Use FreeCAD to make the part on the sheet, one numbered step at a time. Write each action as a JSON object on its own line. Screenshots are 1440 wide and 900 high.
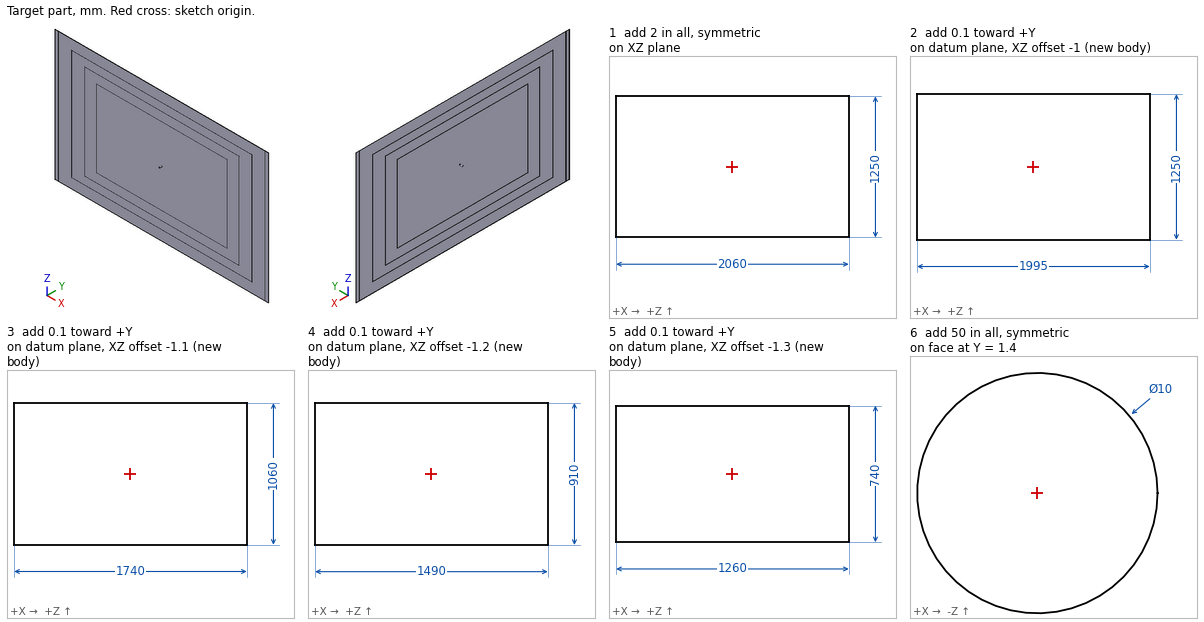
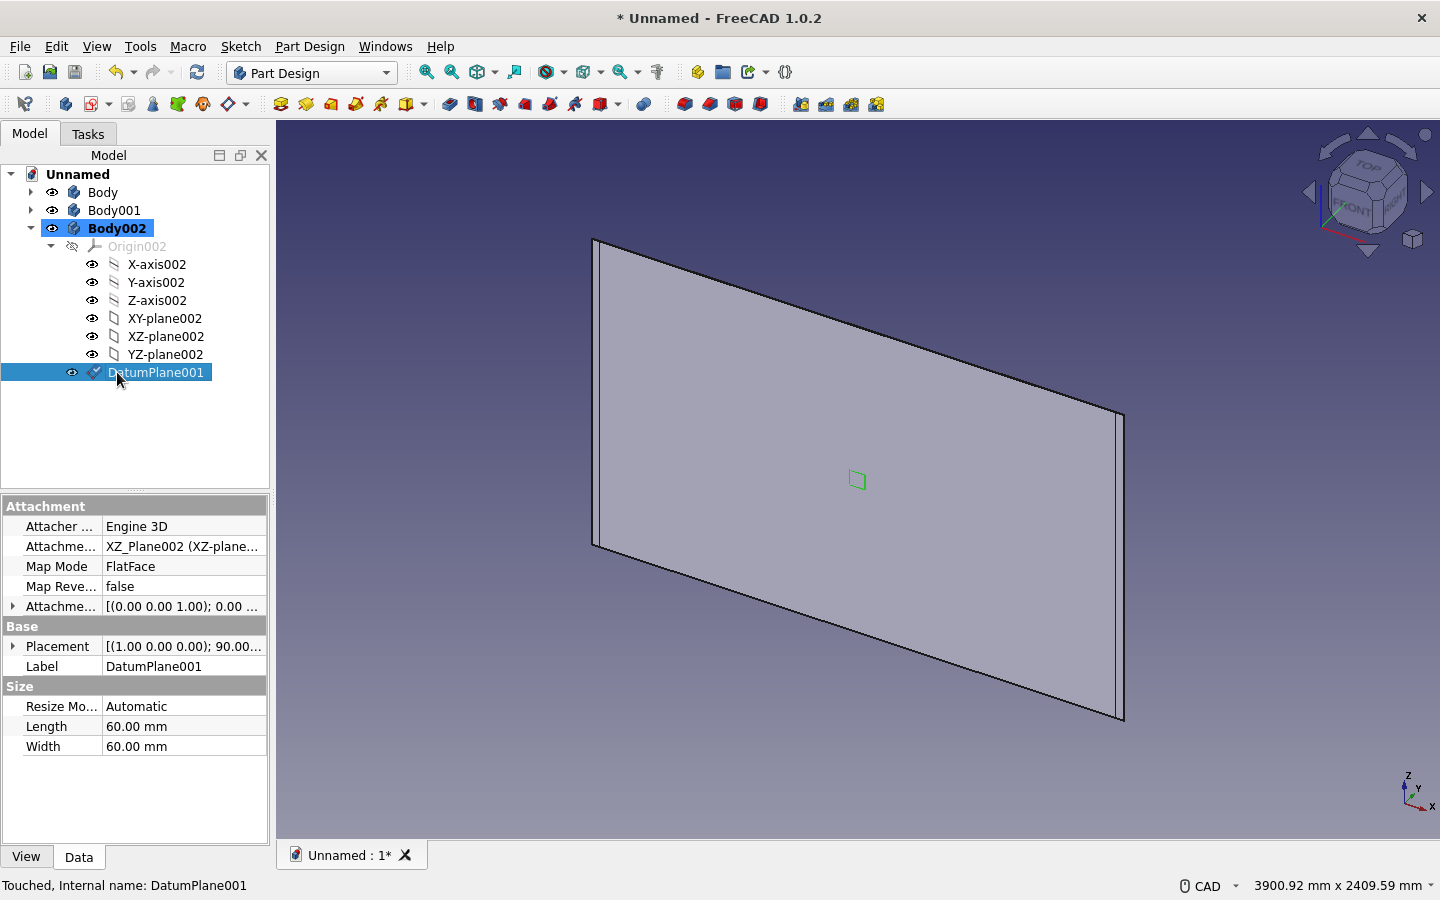
{"action": "left_click", "coordinate": [90, 104]}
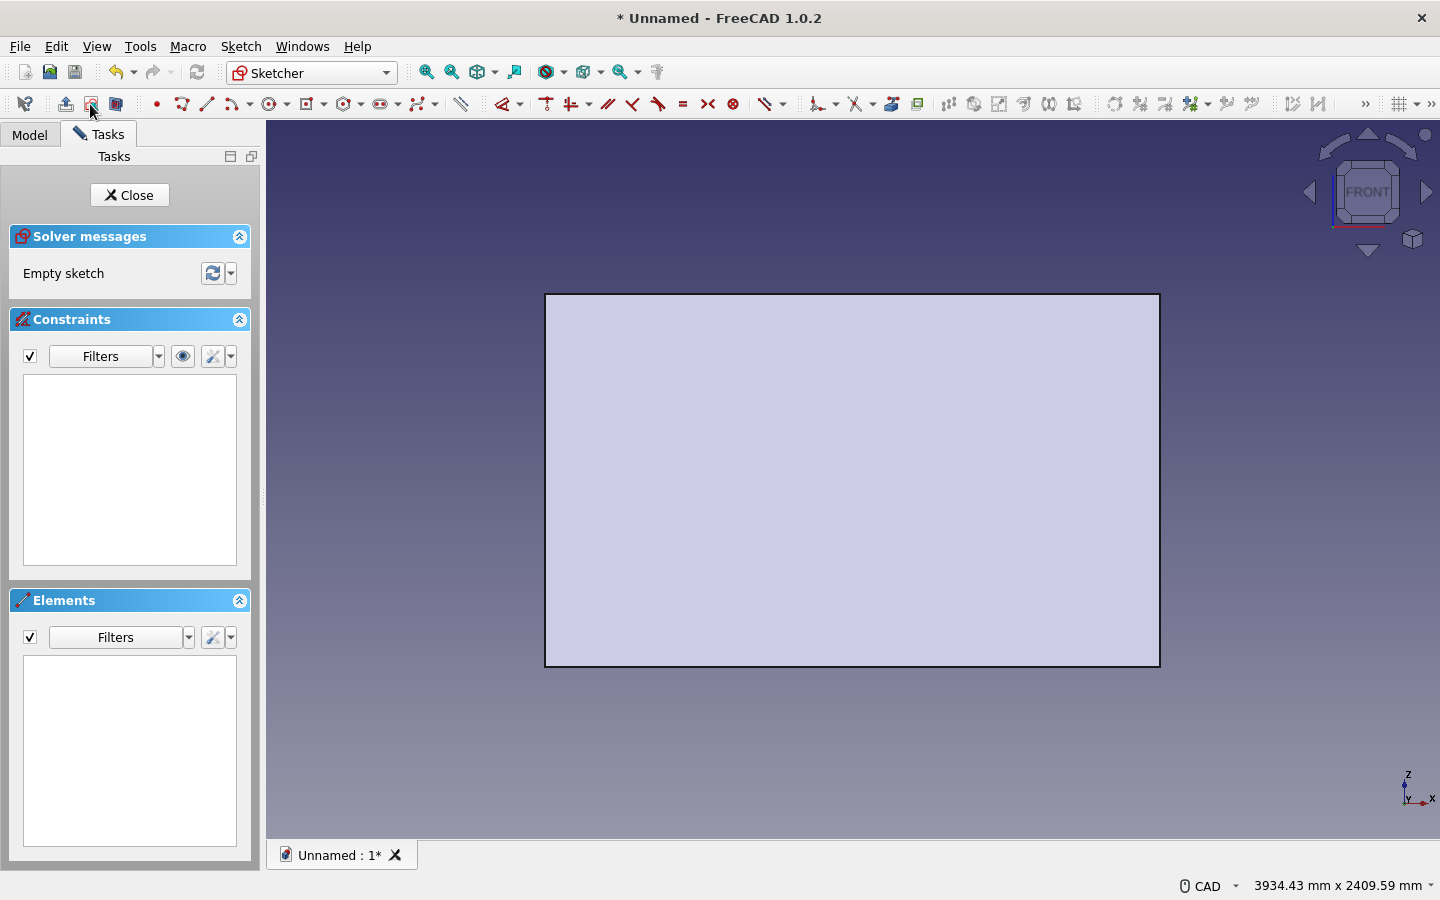
{"action": "left_click", "coordinate": [306, 104]}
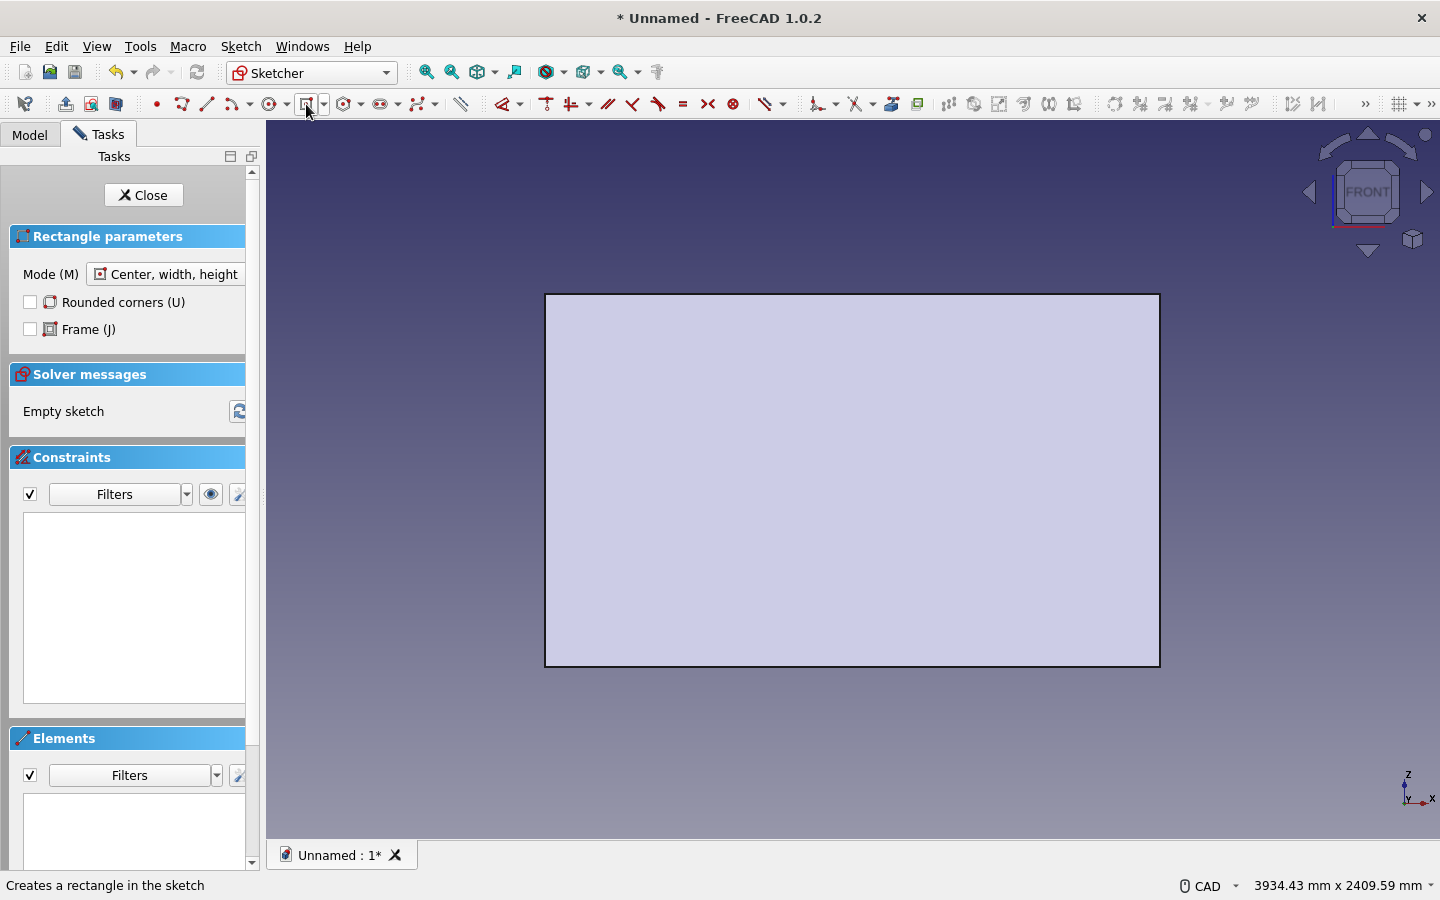
{"action": "left_click", "coordinate": [853, 480]}
{"action": "mouse_move", "coordinate": [1112, 322]}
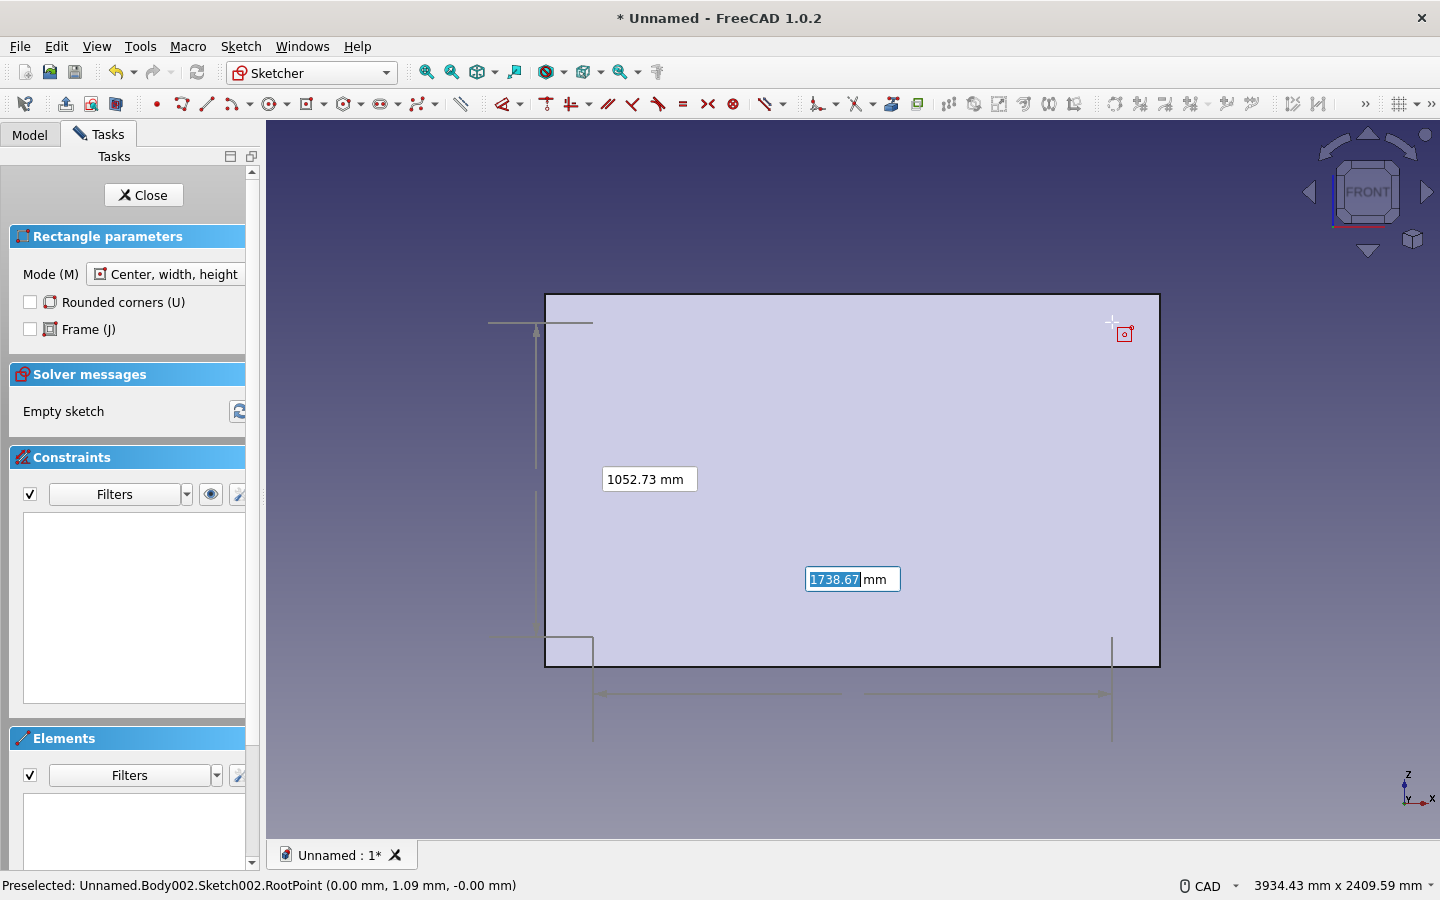
{"action": "type", "text": "1740"}
{"action": "key", "text": "Tab"}
{"action": "type", "text": "1060"}
{"action": "key", "text": "Return"}
{"action": "key", "text": "Escape"}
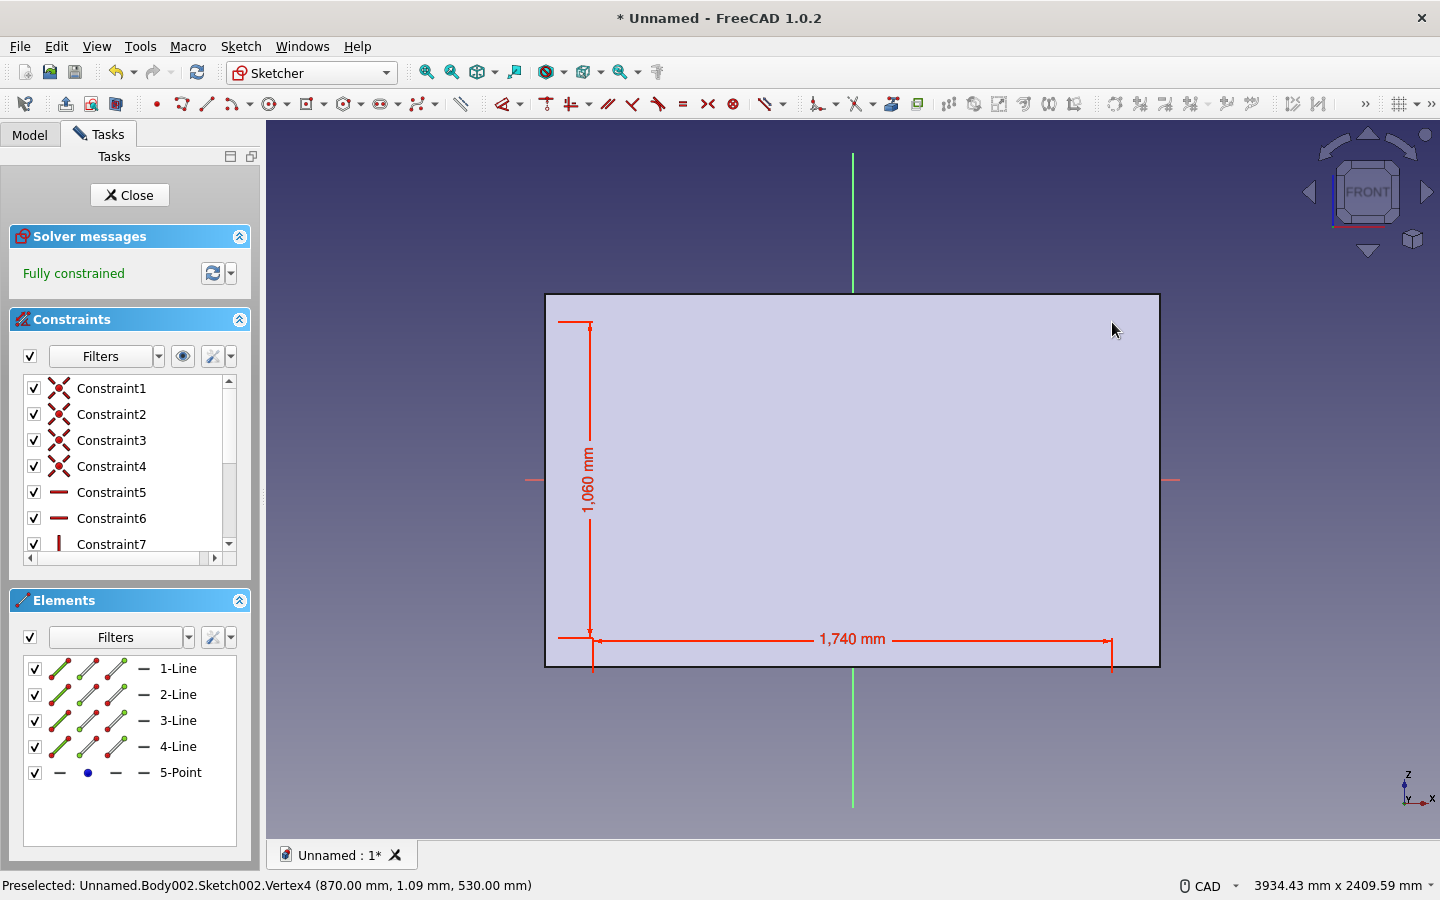
{"action": "left_click", "coordinate": [130, 195]}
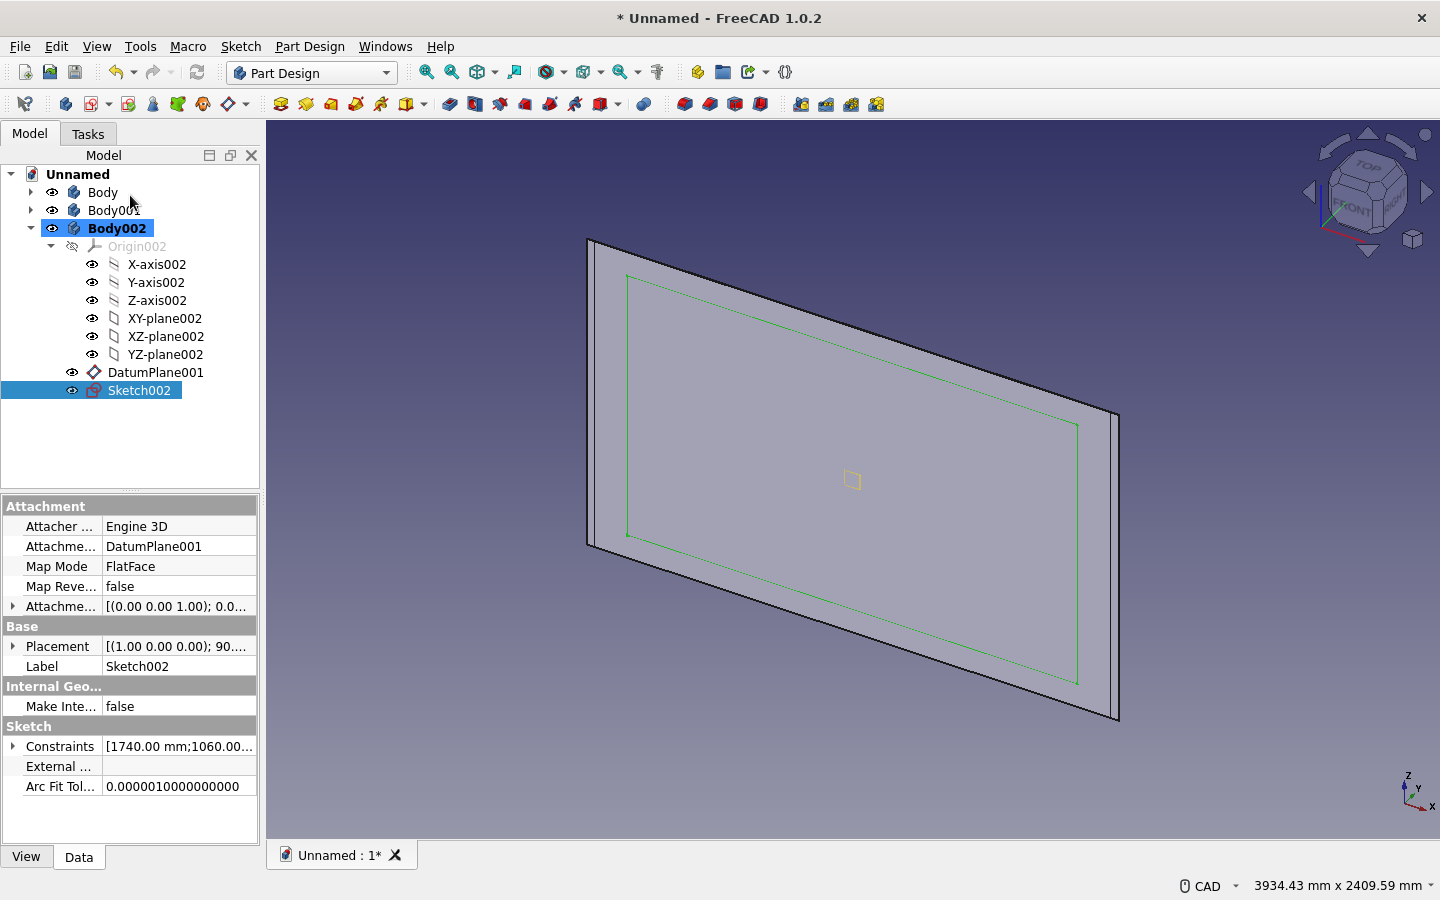
{"action": "left_click", "coordinate": [281, 104]}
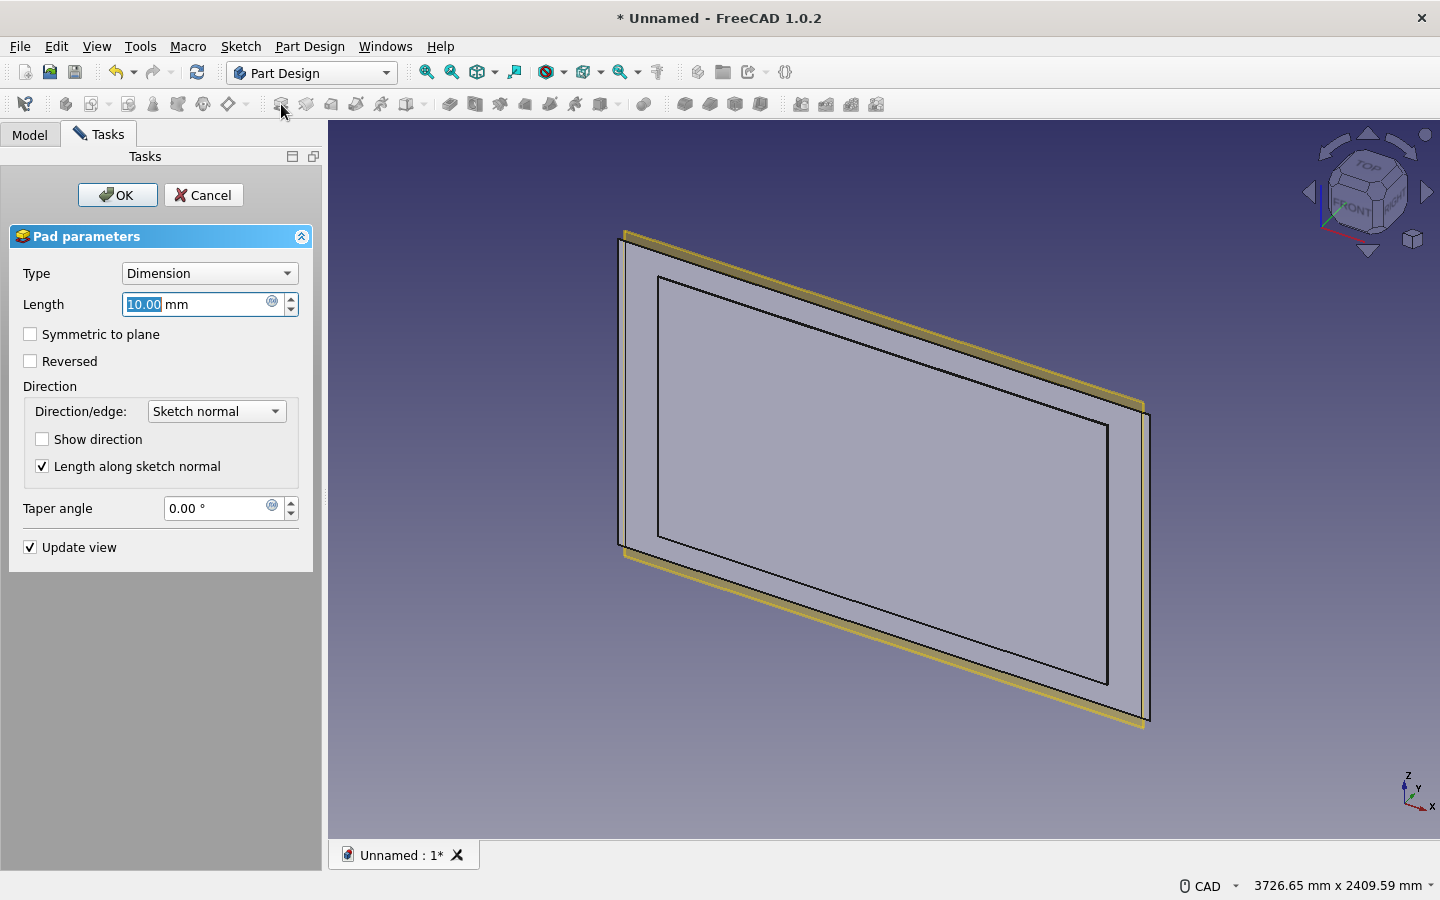
{"action": "type", "text": "0.1"}
{"action": "key", "text": "Tab"}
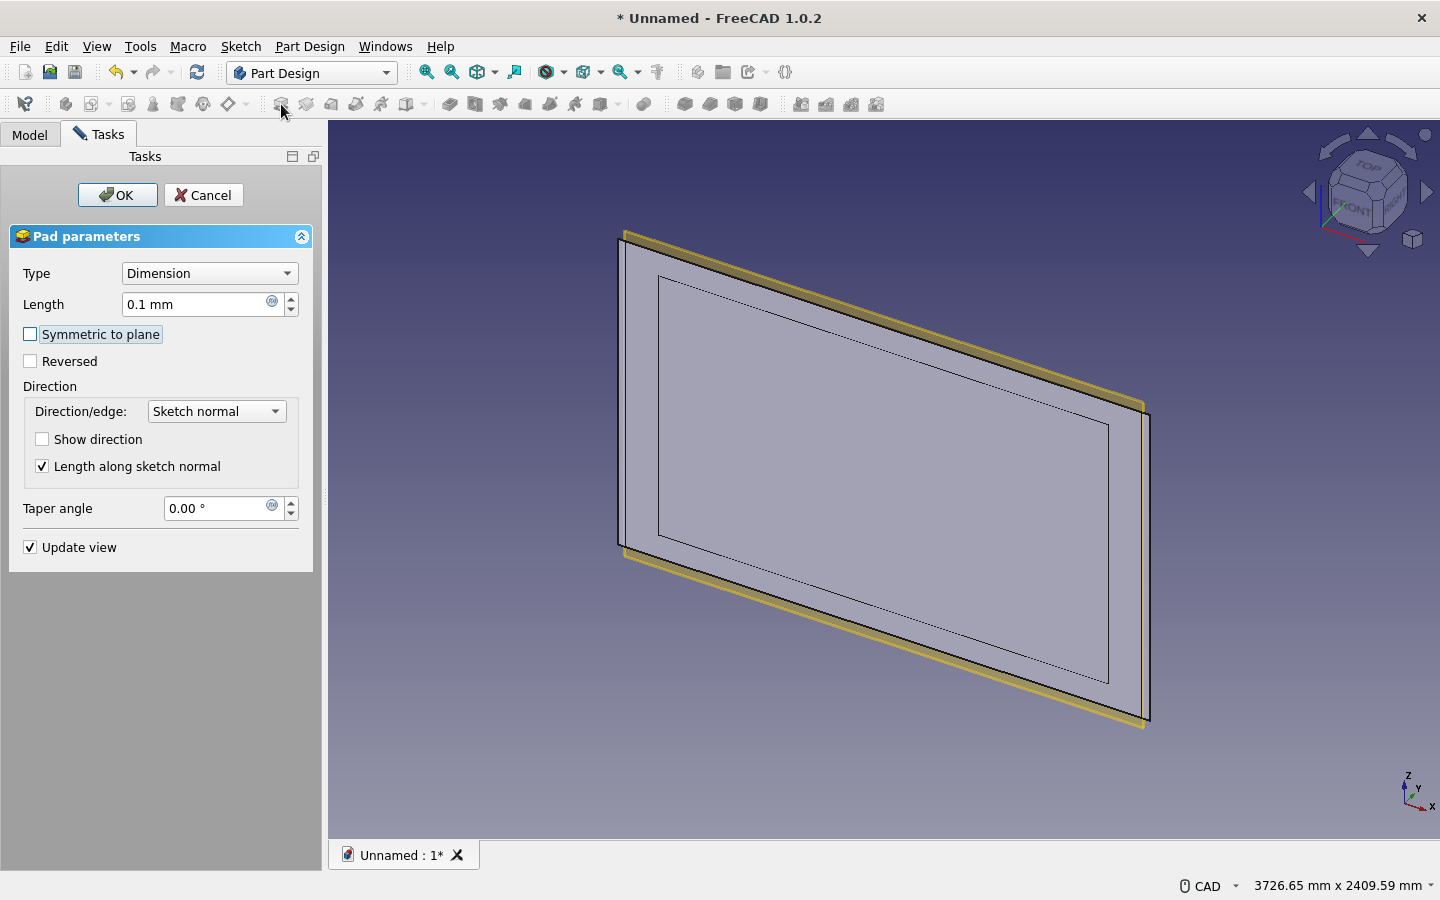
{"action": "left_click", "coordinate": [31, 361]}